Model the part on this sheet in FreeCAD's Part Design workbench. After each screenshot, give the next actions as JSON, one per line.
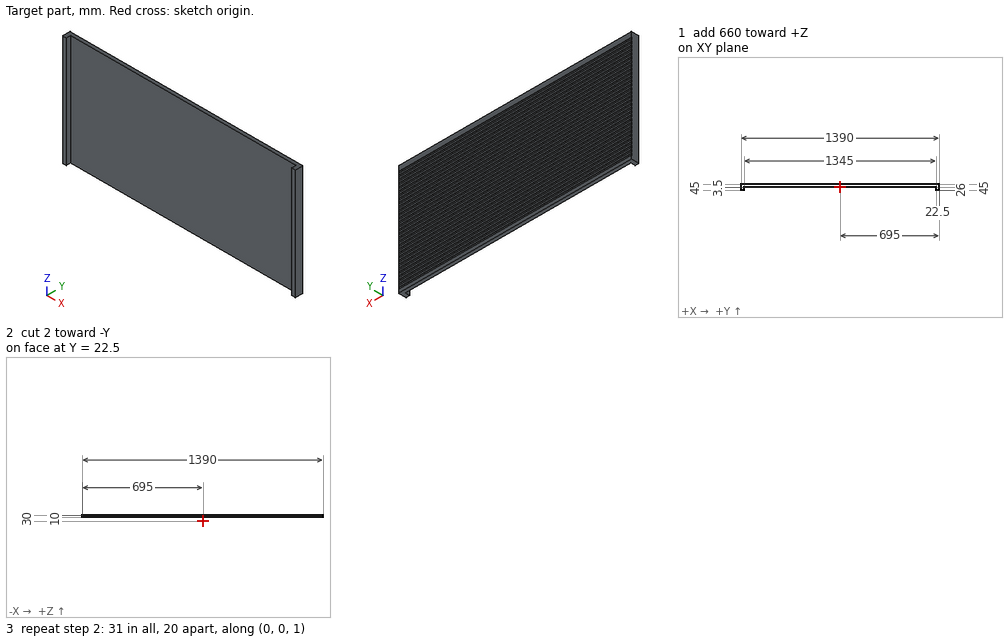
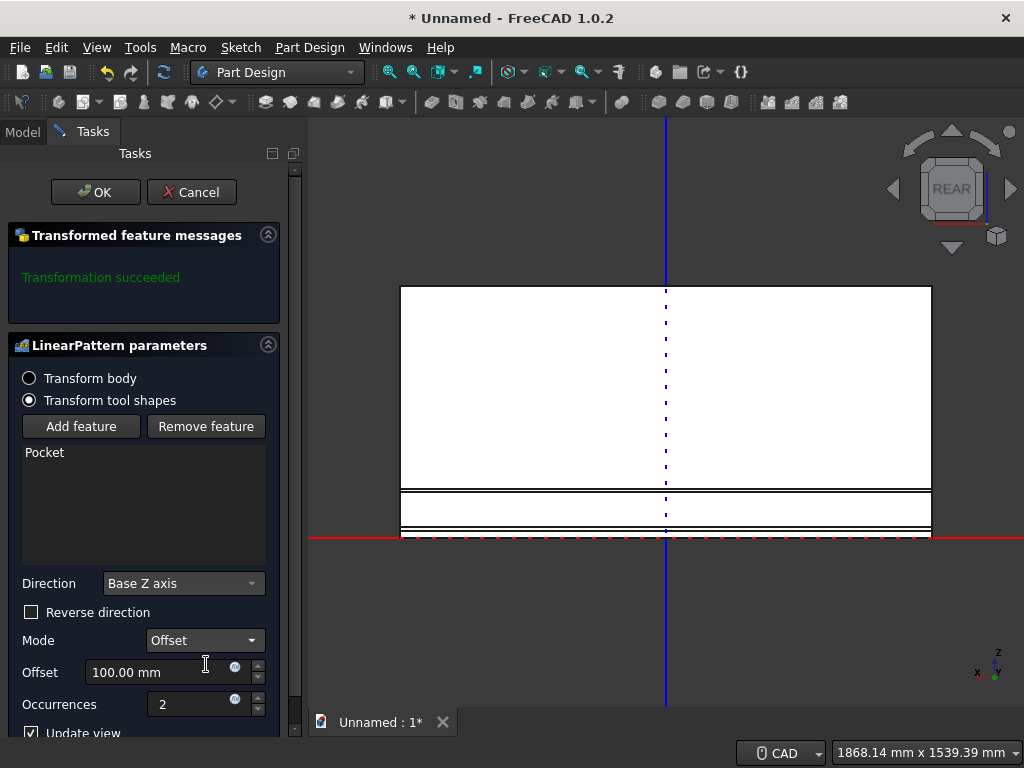
{"action": "triple_click", "coordinate": [168, 672]}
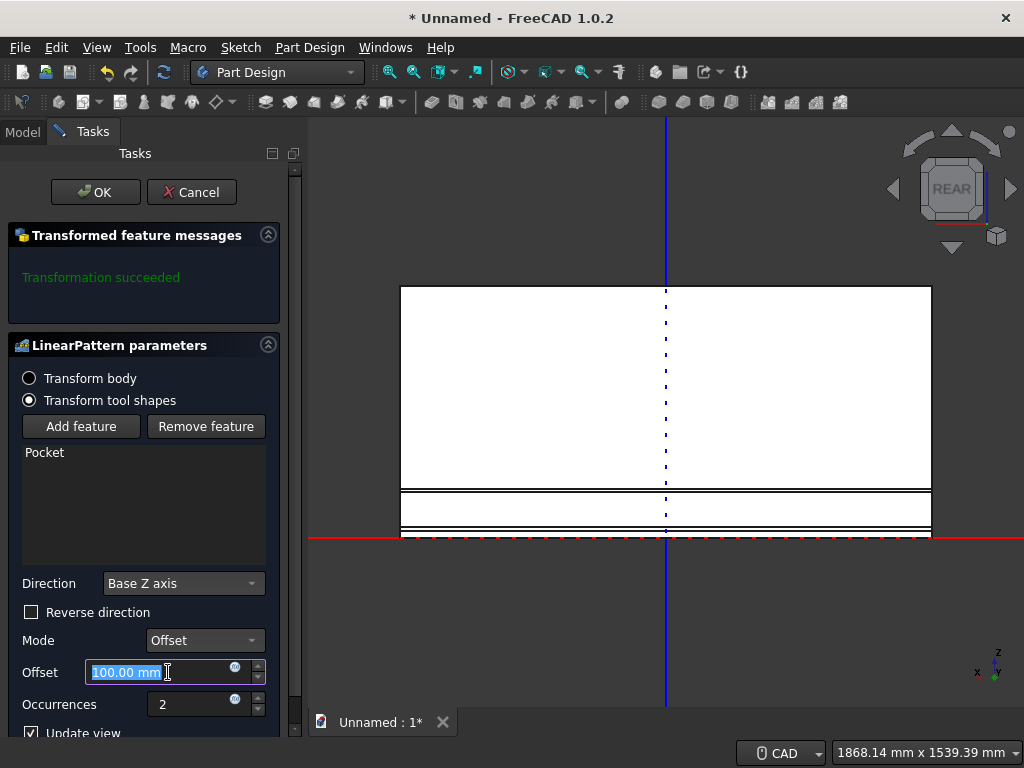
{"action": "type", "text": "20"}
{"action": "key", "text": "Tab"}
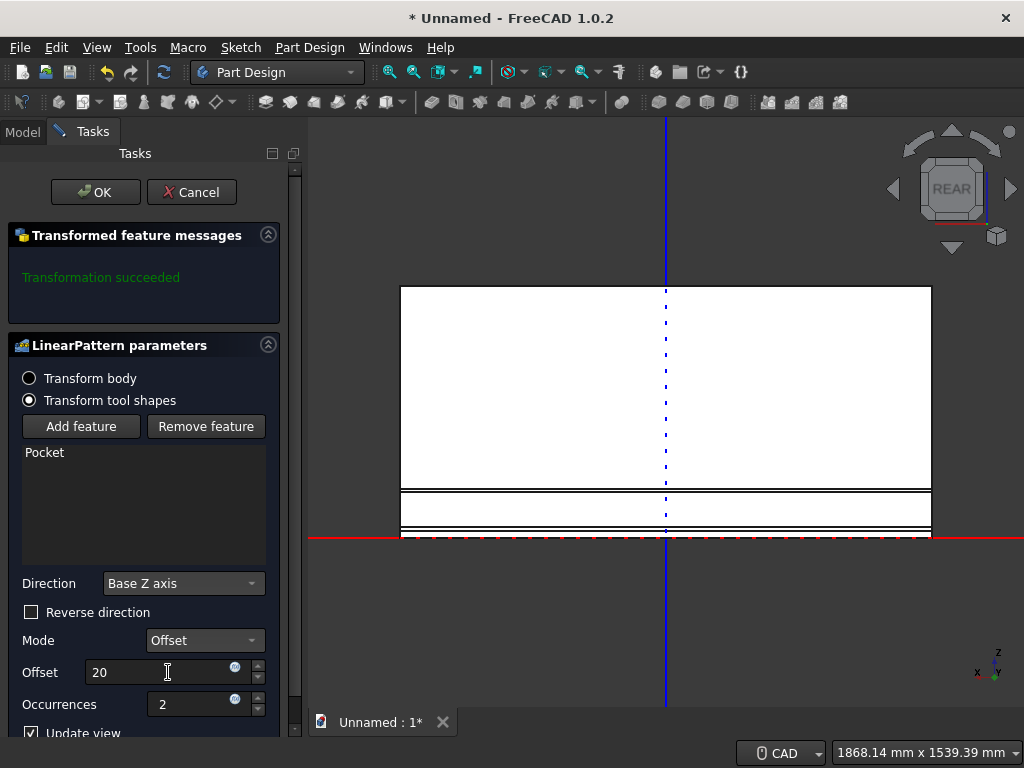
{"action": "triple_click", "coordinate": [198, 704]}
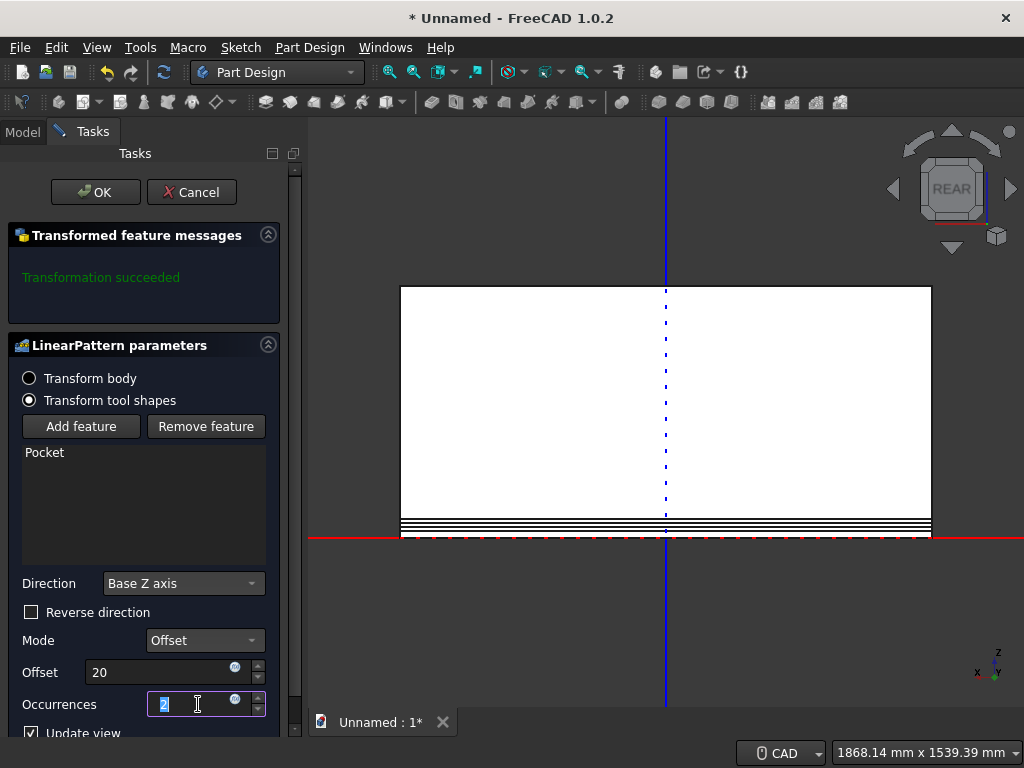
{"action": "type", "text": "31"}
{"action": "key", "text": "Tab"}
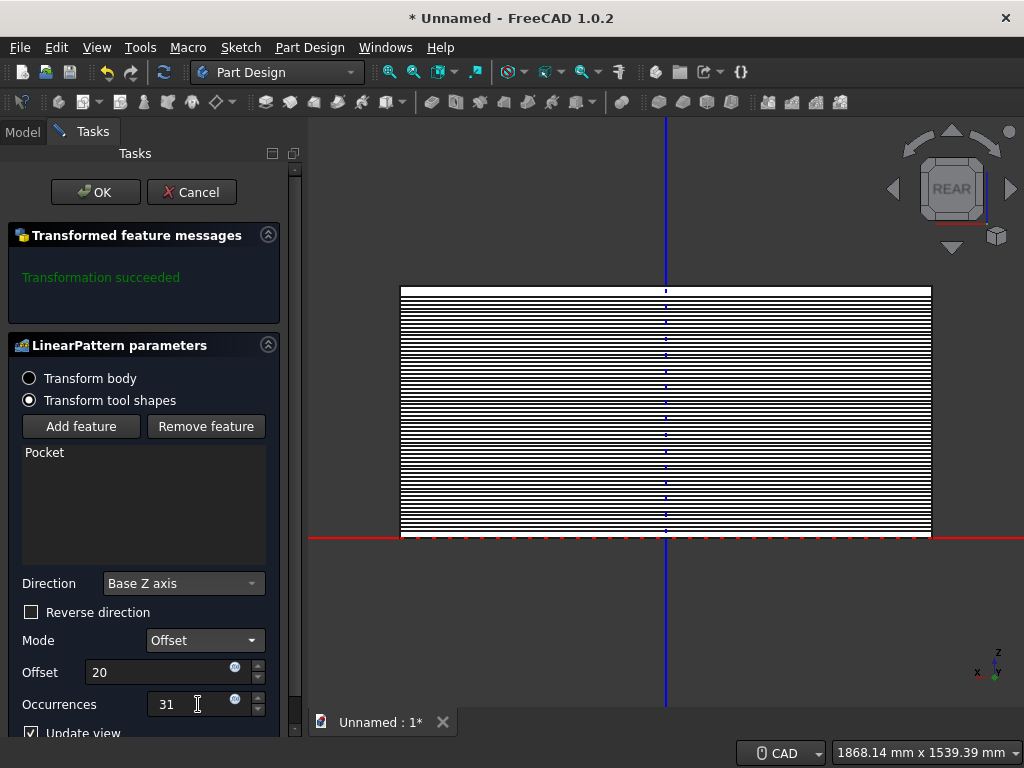
{"action": "left_click", "coordinate": [96, 192]}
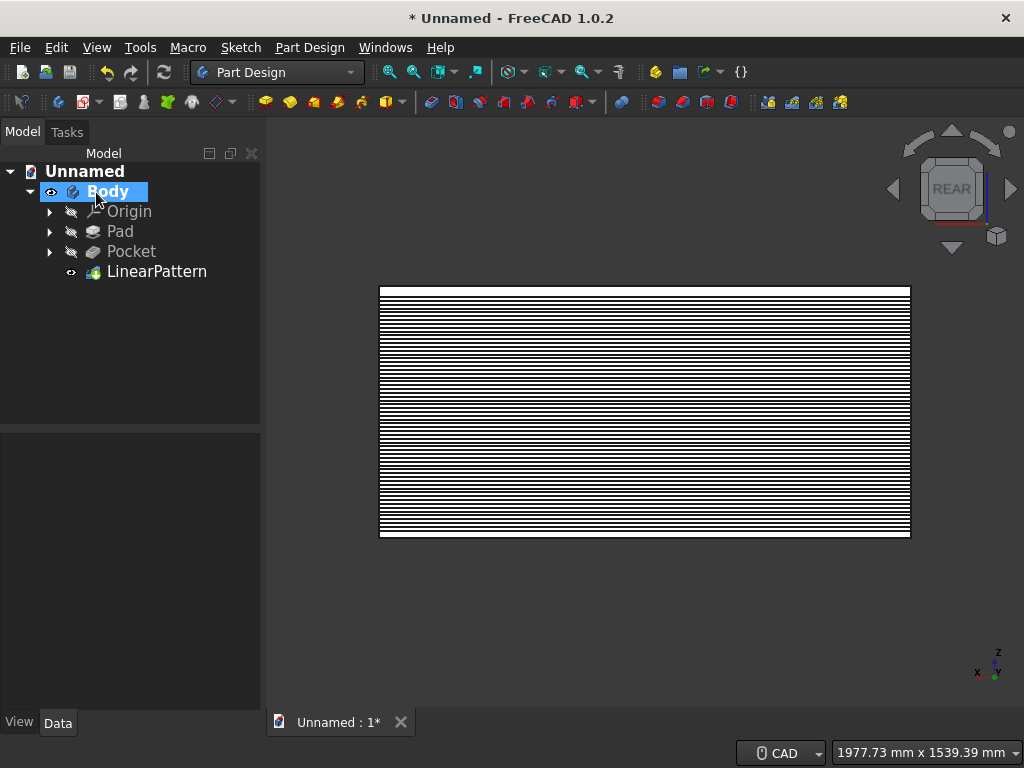
{"action": "key", "text": "0"}